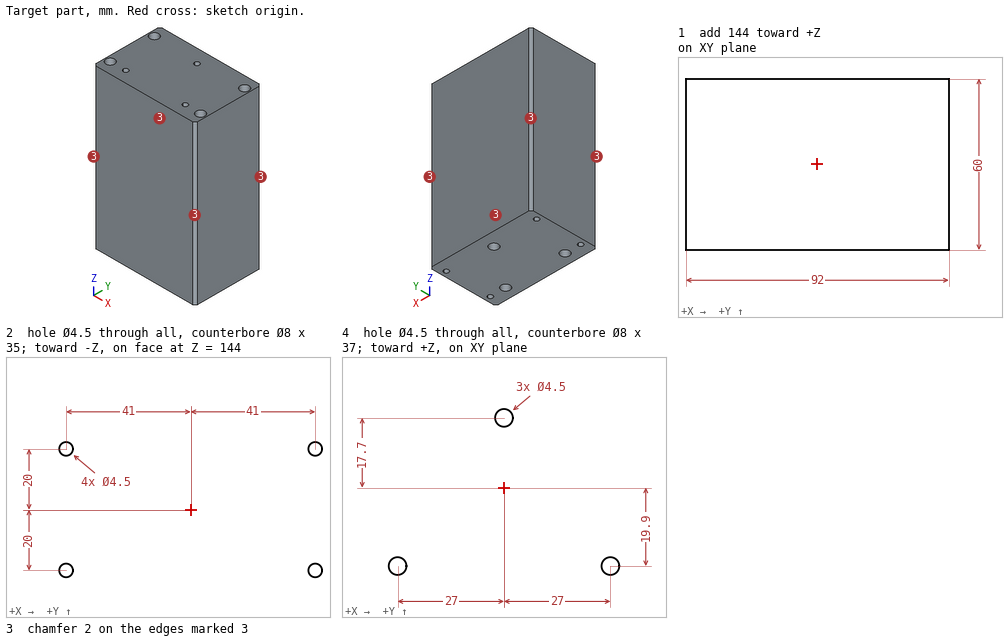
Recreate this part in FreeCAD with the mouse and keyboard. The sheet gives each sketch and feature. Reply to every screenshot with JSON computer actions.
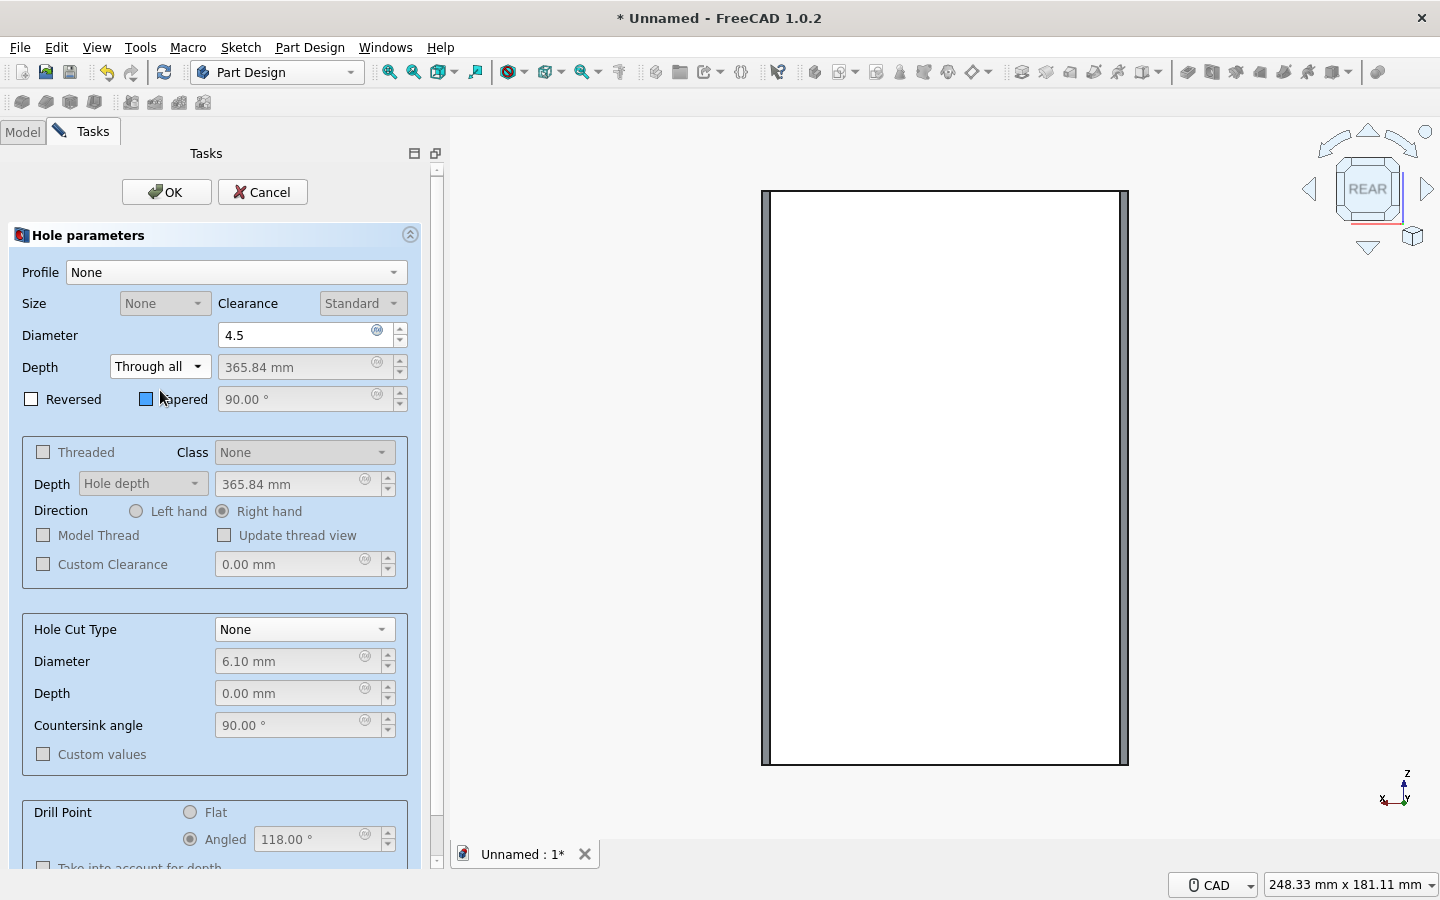
{"action": "left_click", "coordinate": [30, 399]}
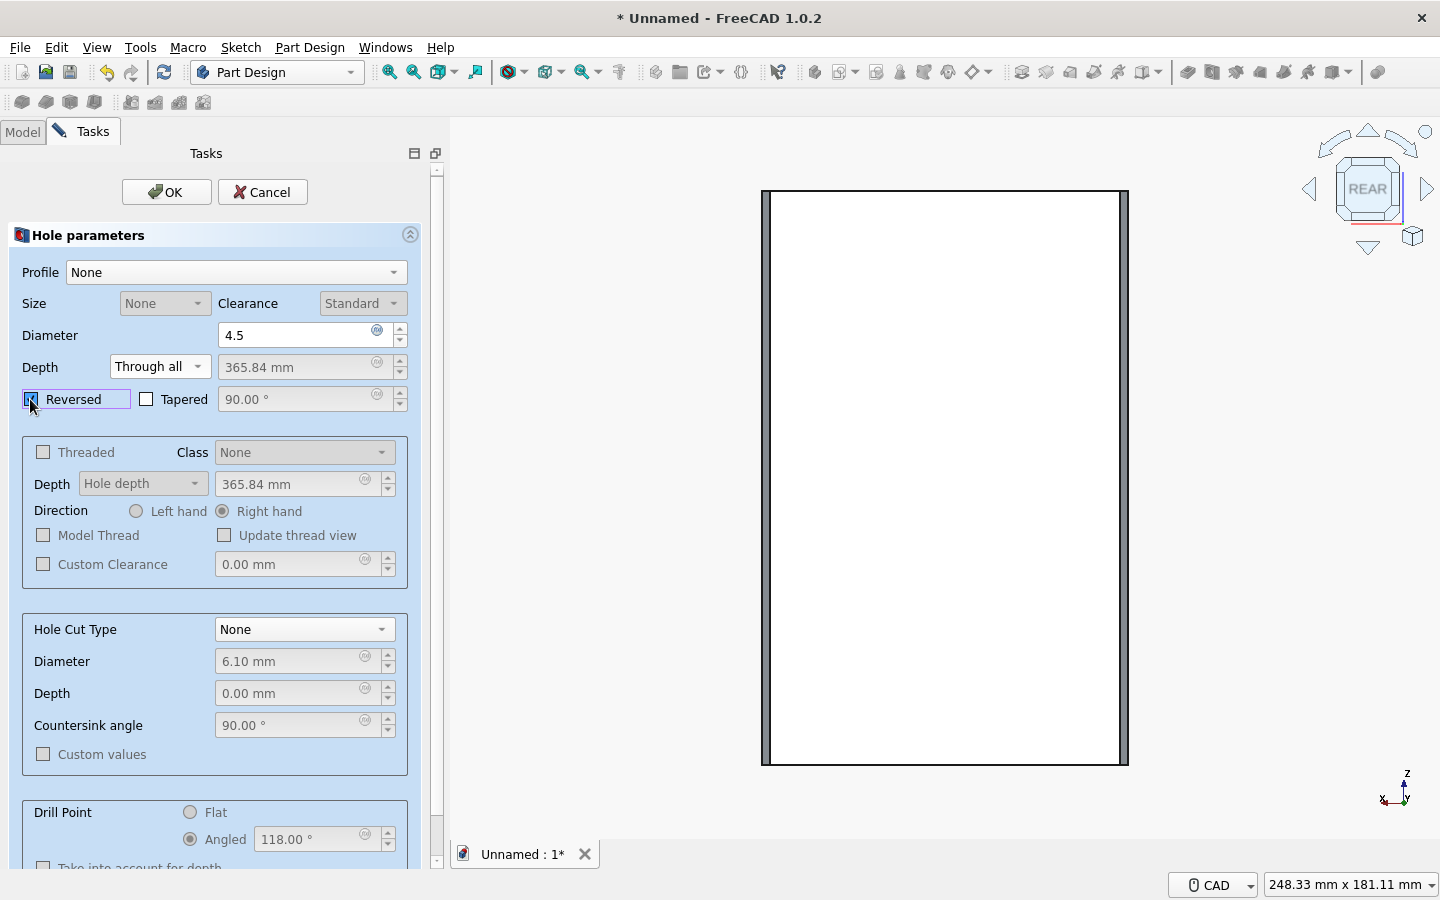
{"action": "left_click", "coordinate": [306, 630]}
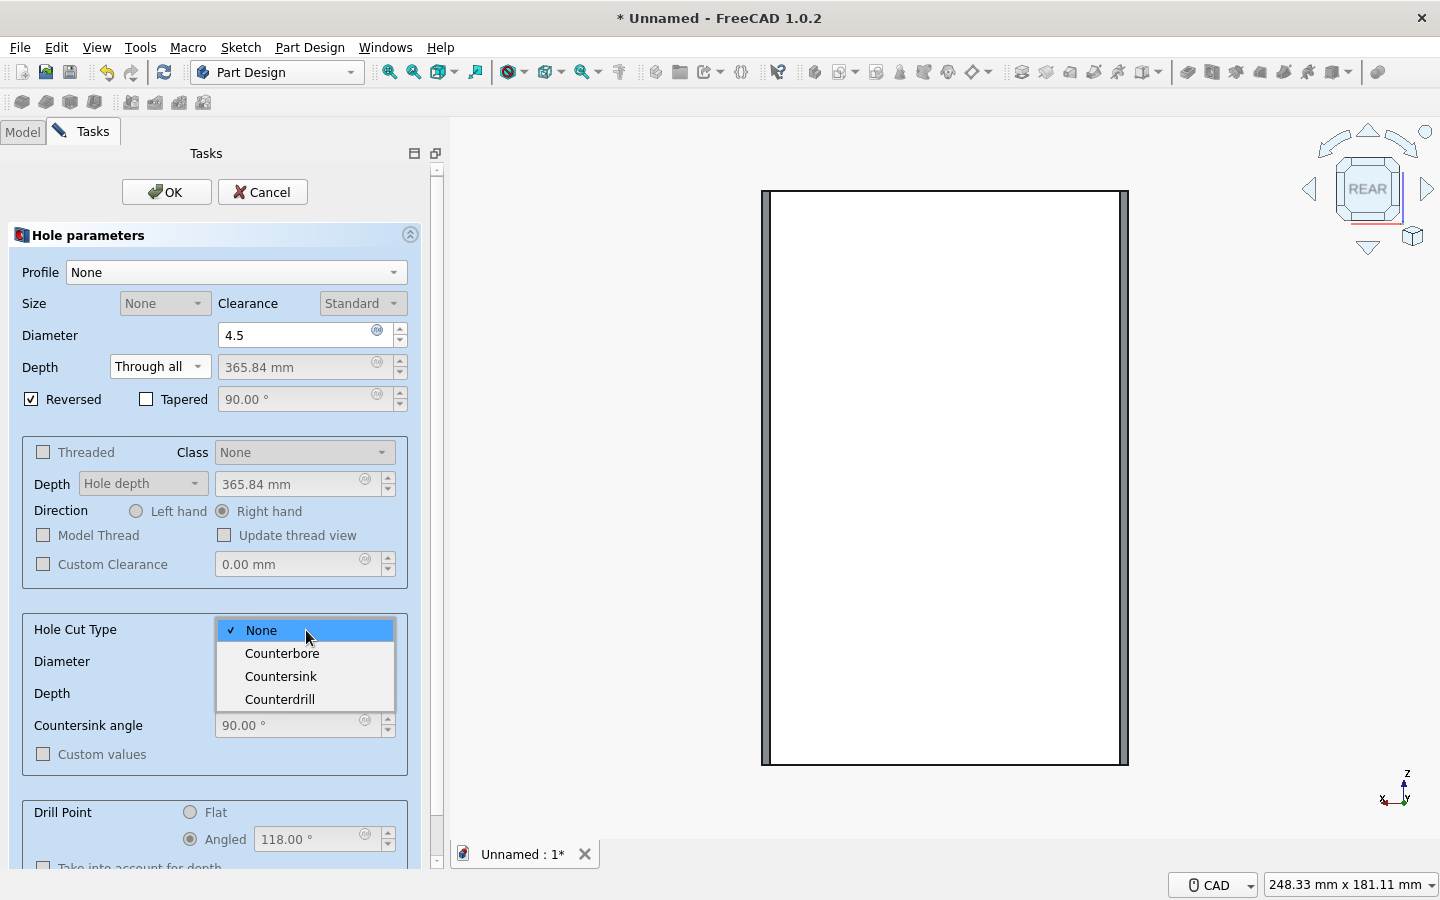
{"action": "left_click", "coordinate": [304, 654]}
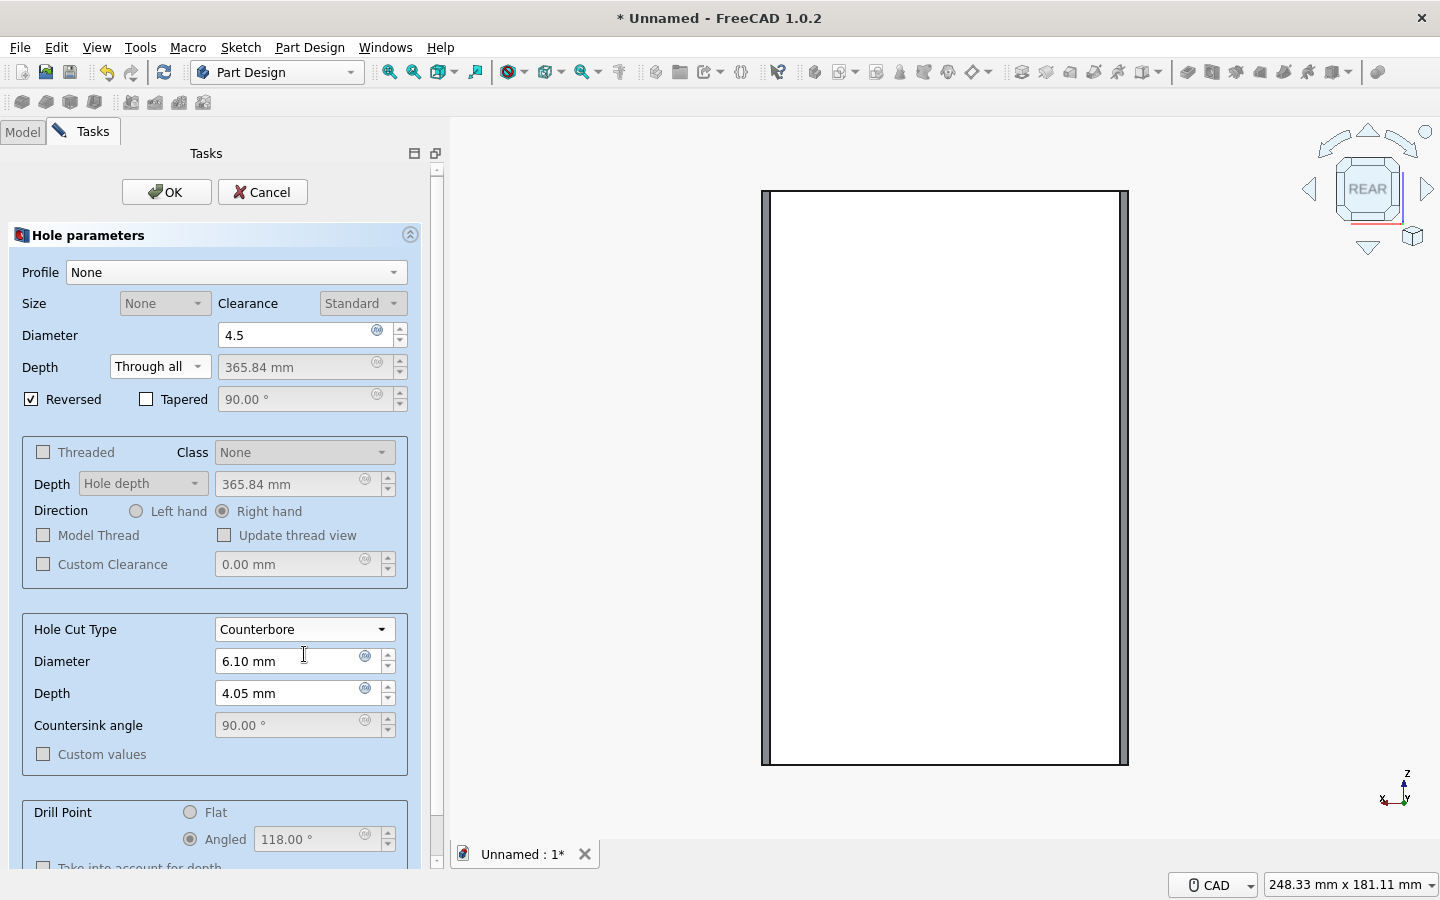
{"action": "triple_click", "coordinate": [298, 661]}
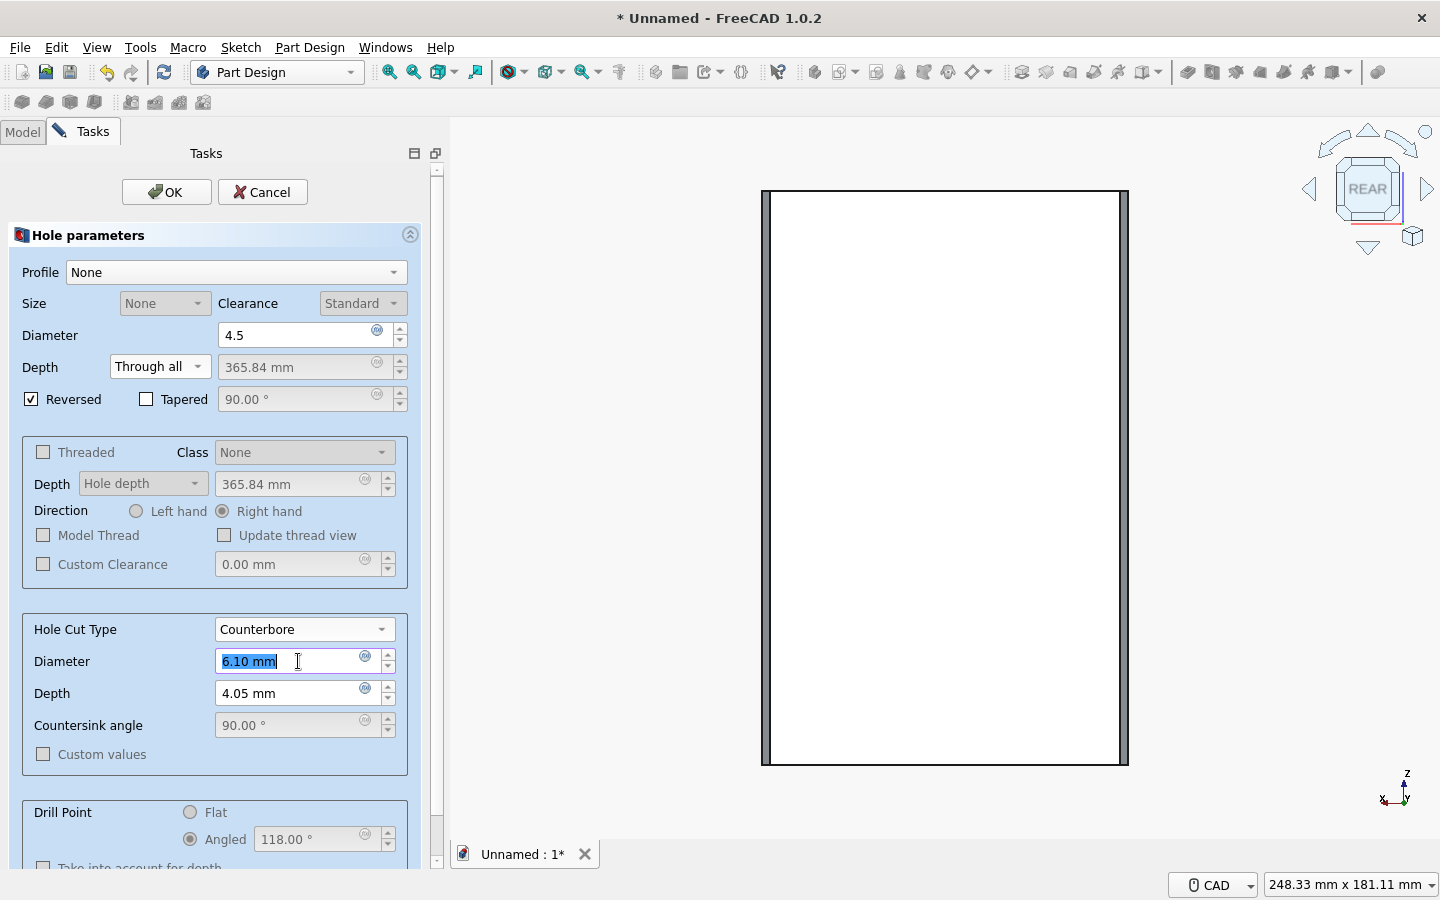
{"action": "type", "text": "8"}
{"action": "key", "text": "Tab"}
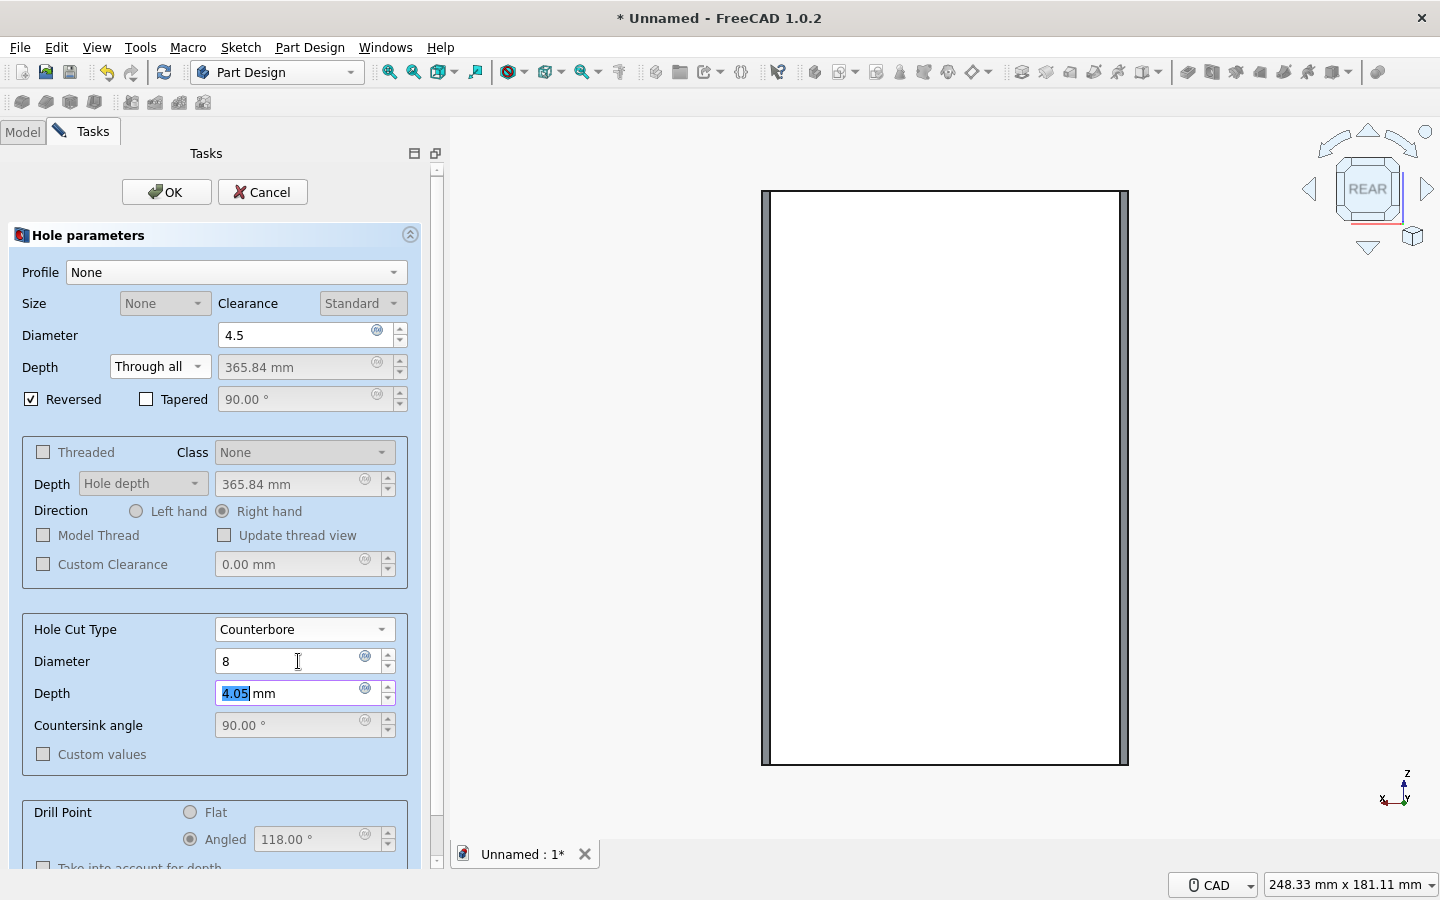
{"action": "type", "text": "37"}
{"action": "key", "text": "Tab"}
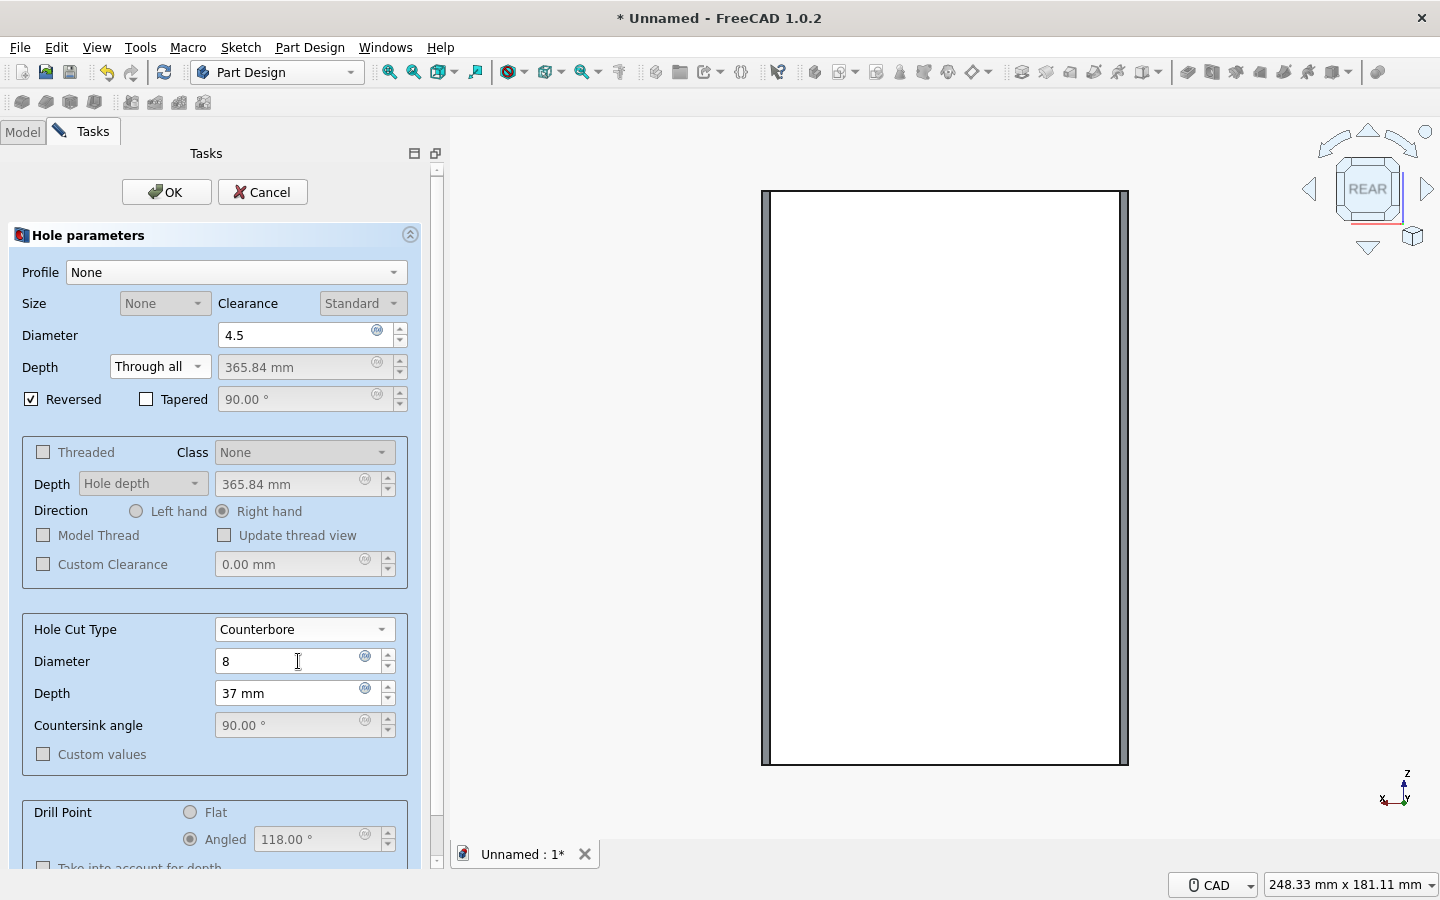
{"action": "left_click", "coordinate": [167, 192]}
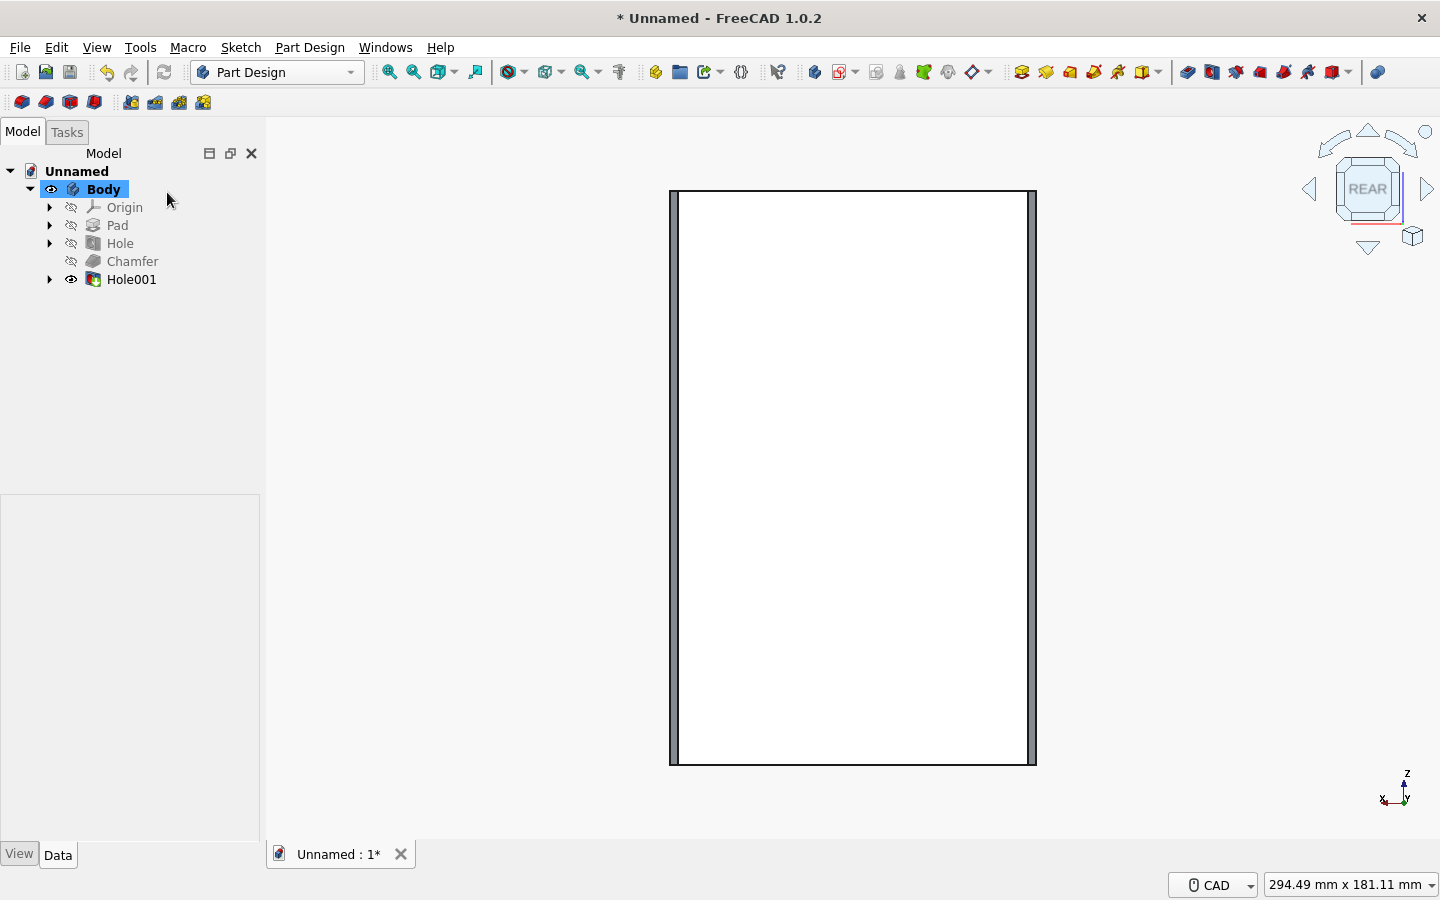
{"action": "key", "text": "0"}